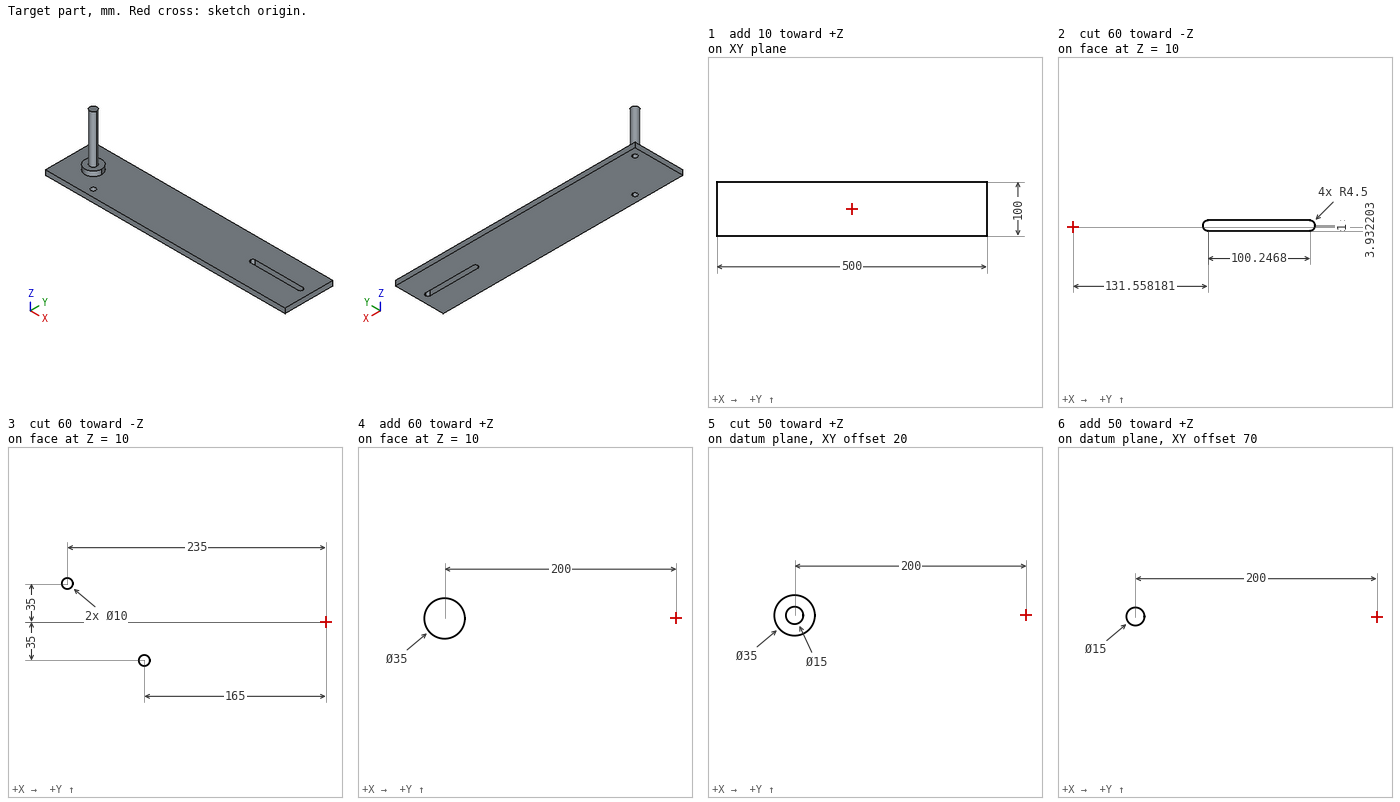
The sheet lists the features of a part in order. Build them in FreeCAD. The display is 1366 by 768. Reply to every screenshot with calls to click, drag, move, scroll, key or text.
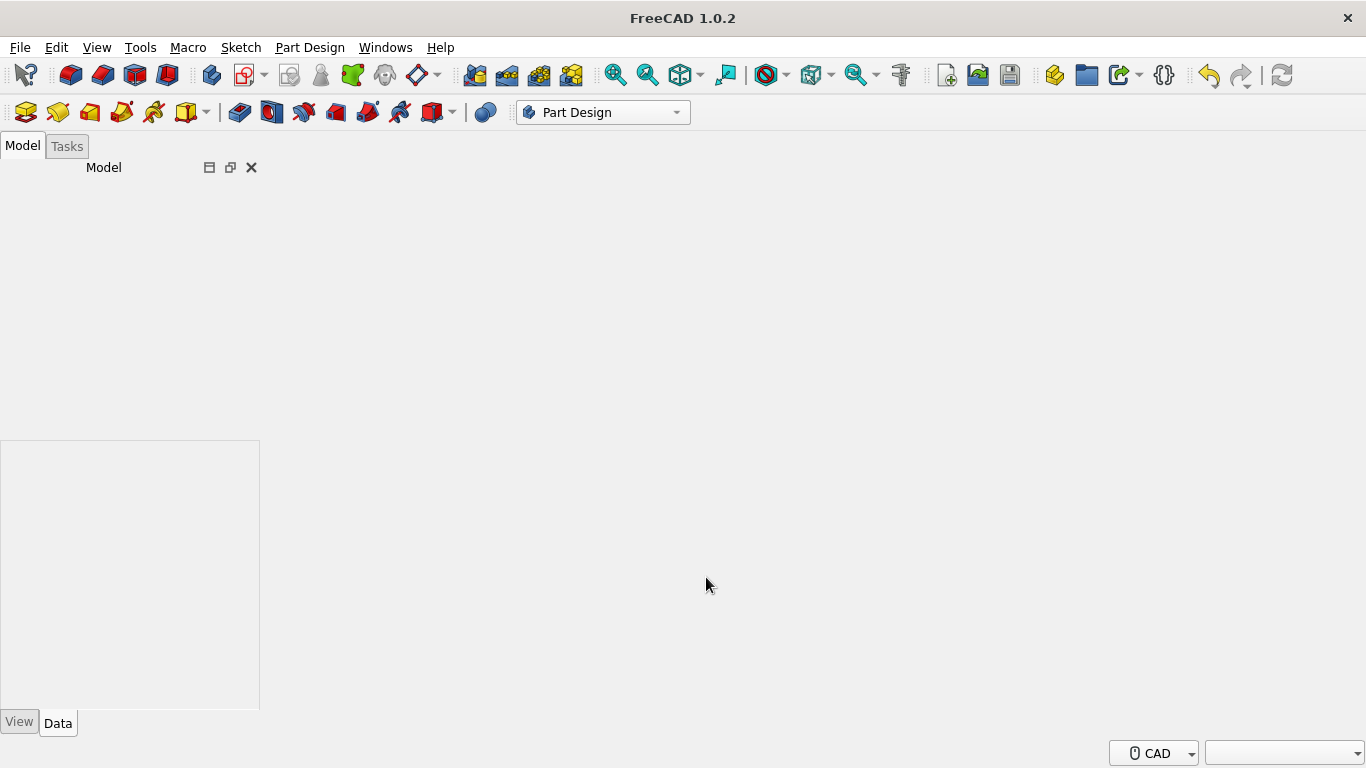
key(ctrl+n)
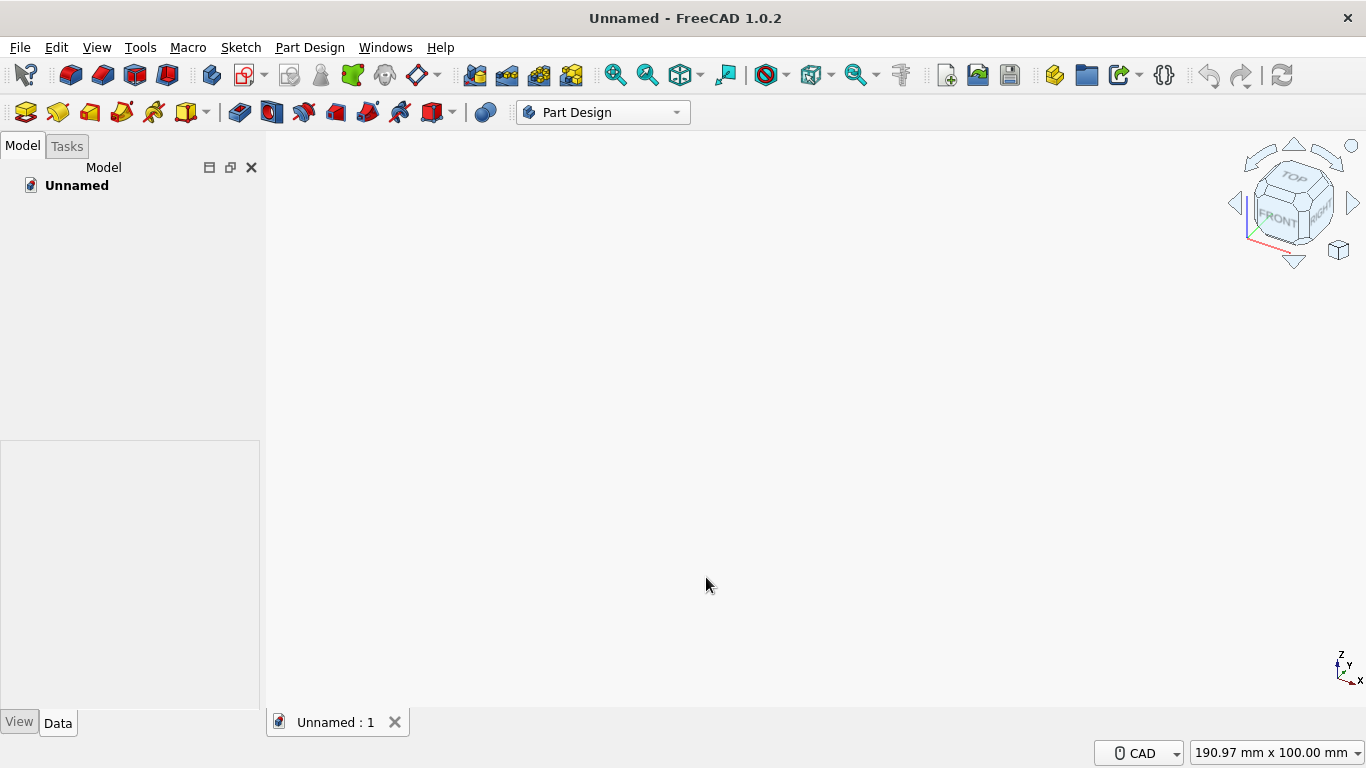
click(244, 76)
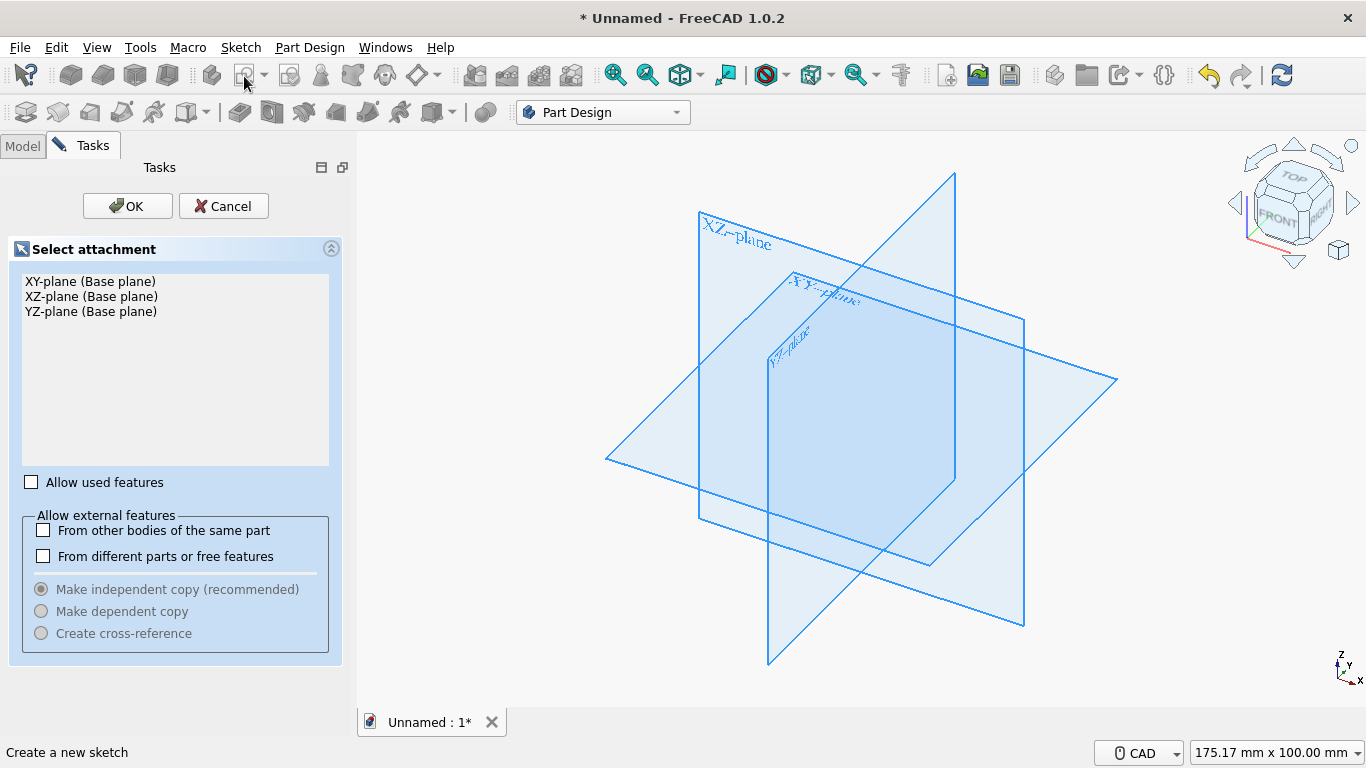
click(82, 282)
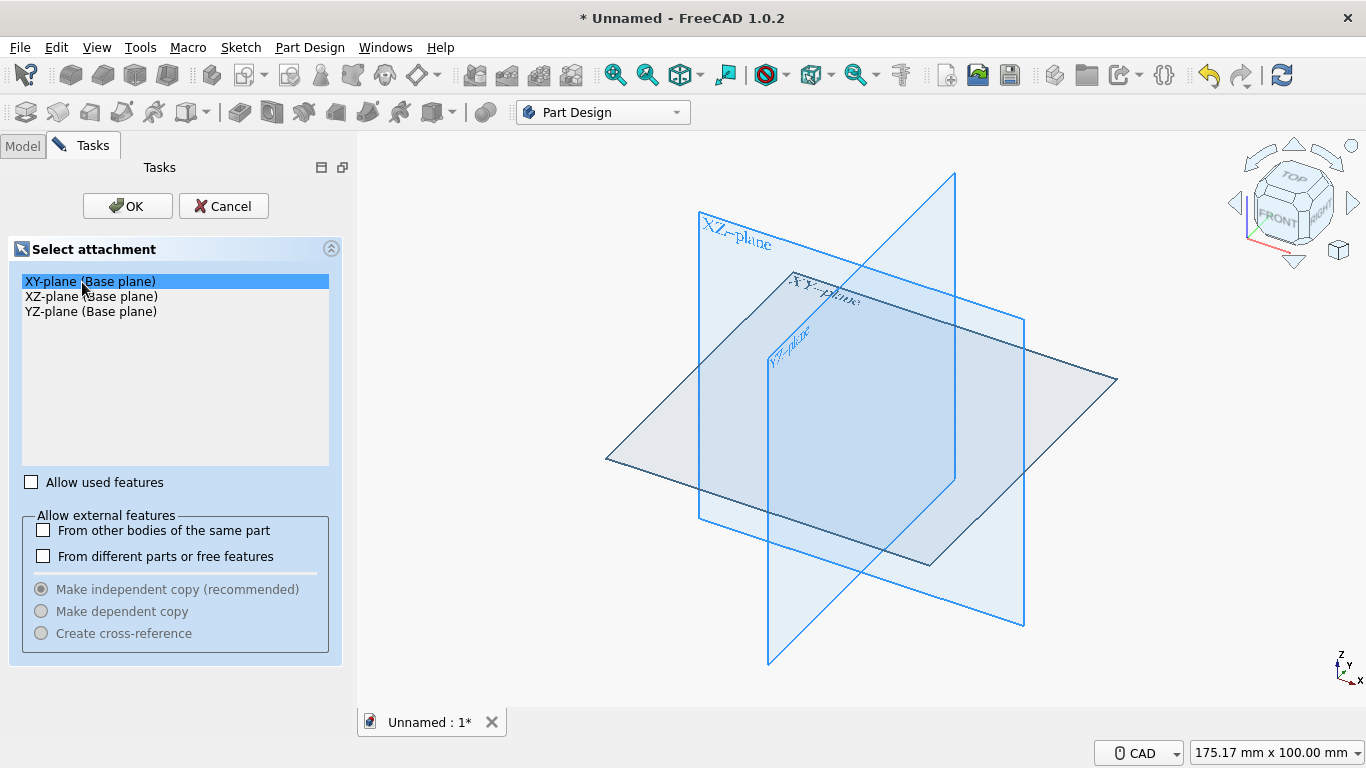
click(128, 206)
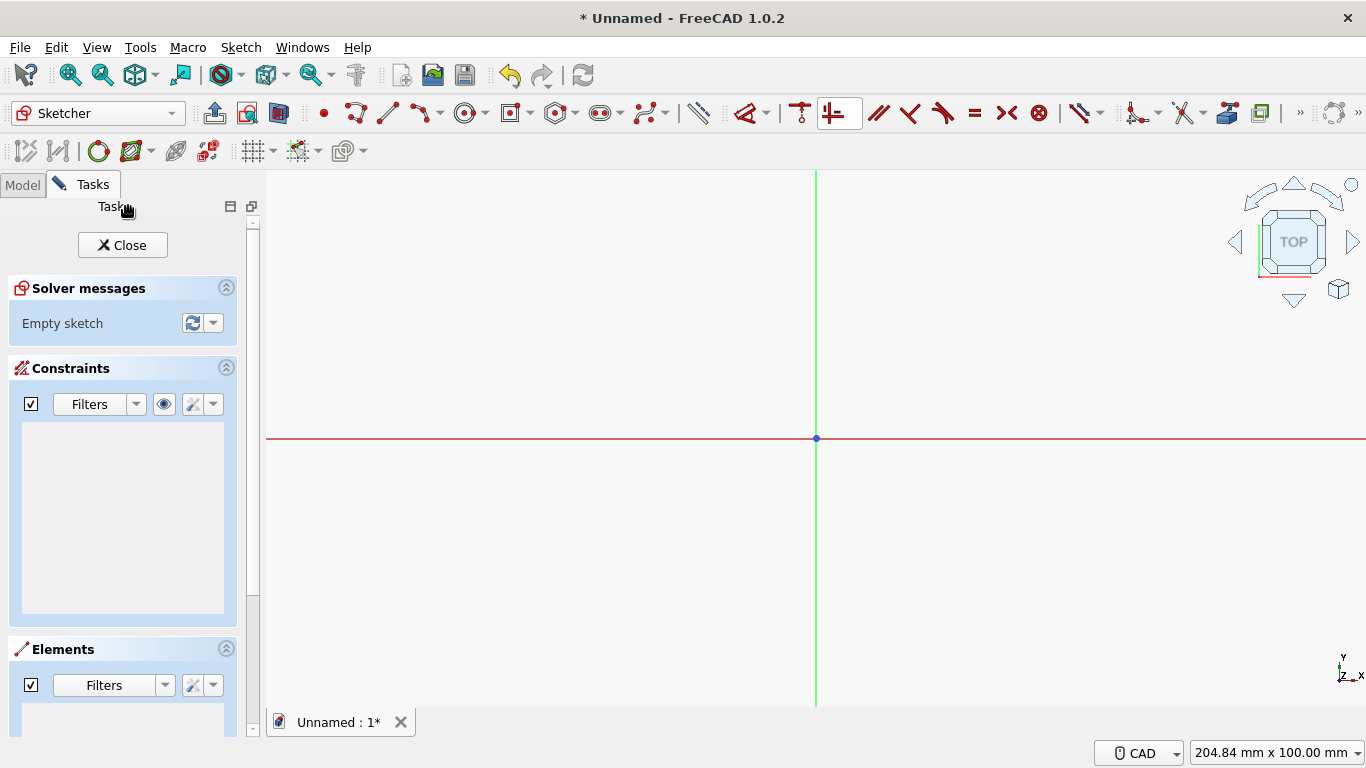
scroll(725, 438, down, 7)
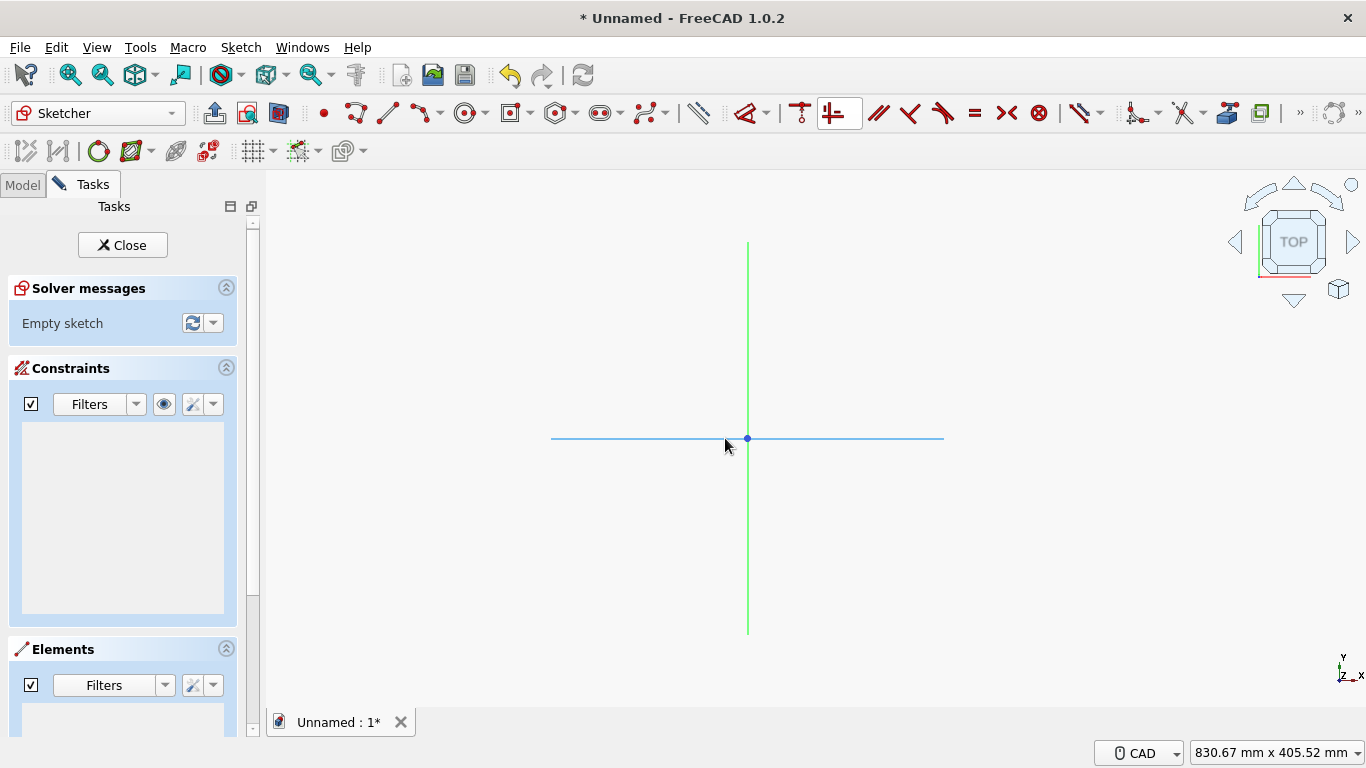
key(g)
key(v)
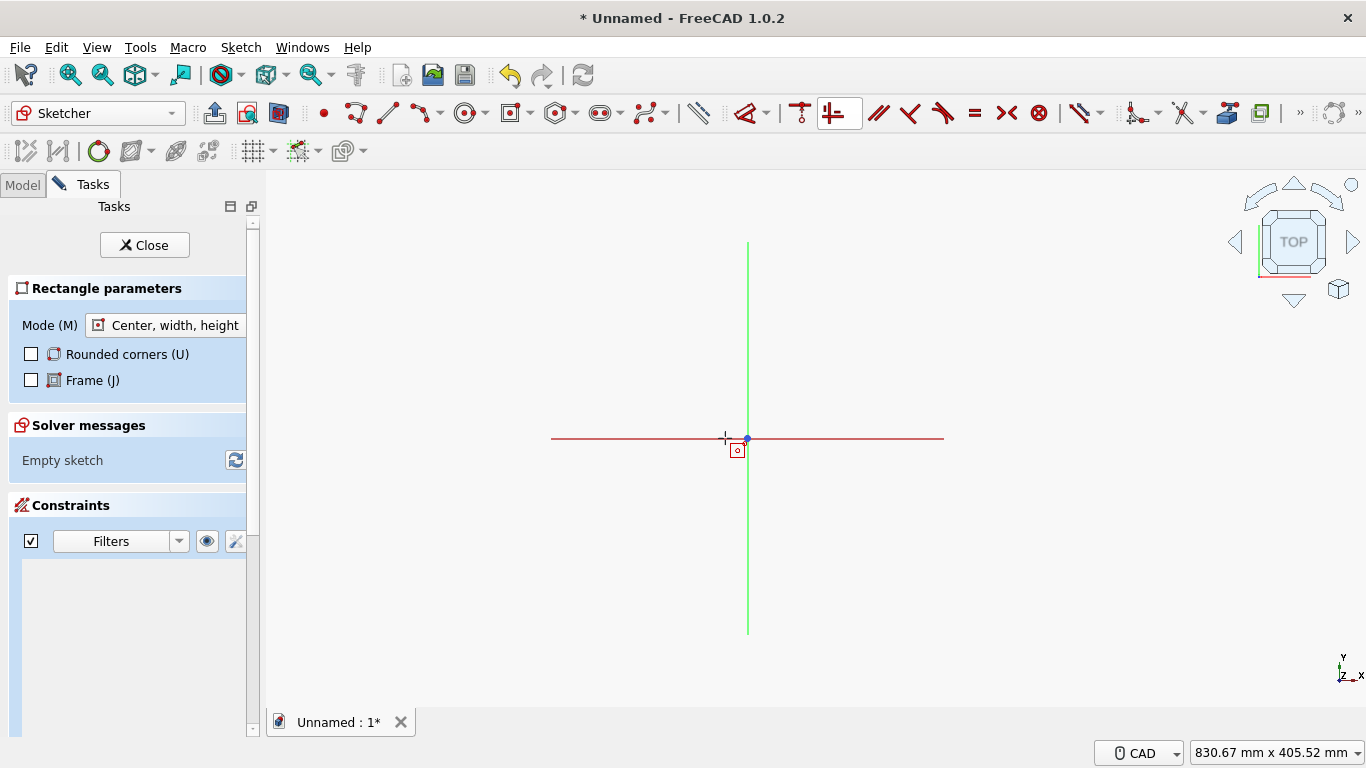
click(748, 438)
move(1079, 372)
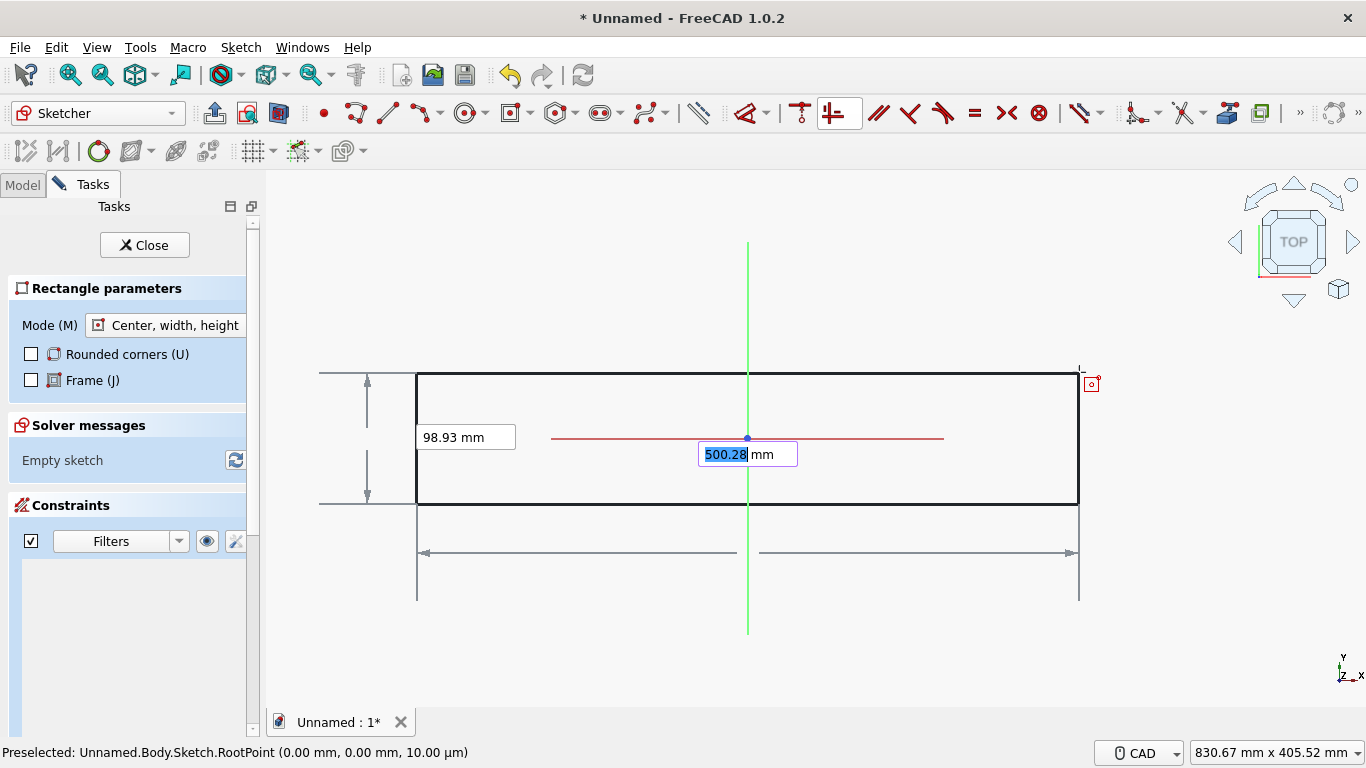
text(500)
key(Tab)
text(100)
key(Return)
key(Escape)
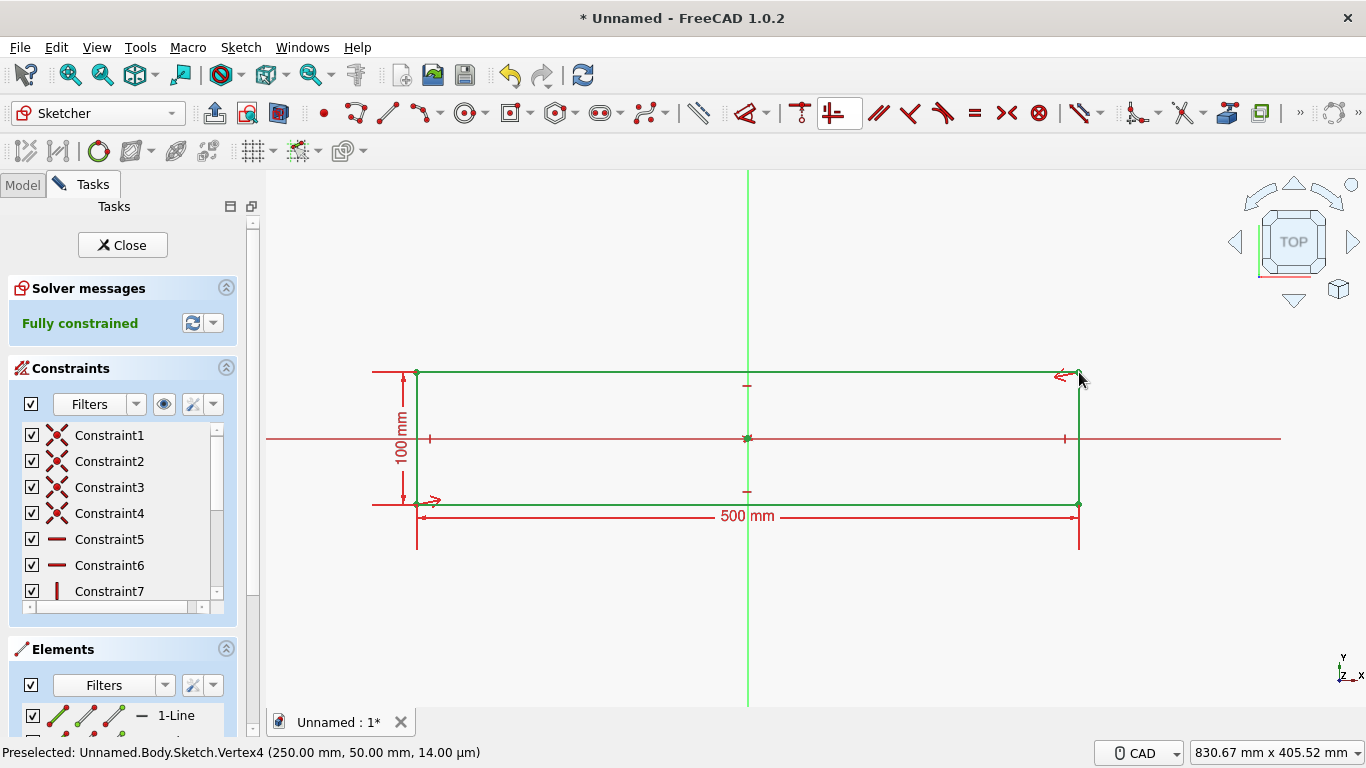
click(123, 245)